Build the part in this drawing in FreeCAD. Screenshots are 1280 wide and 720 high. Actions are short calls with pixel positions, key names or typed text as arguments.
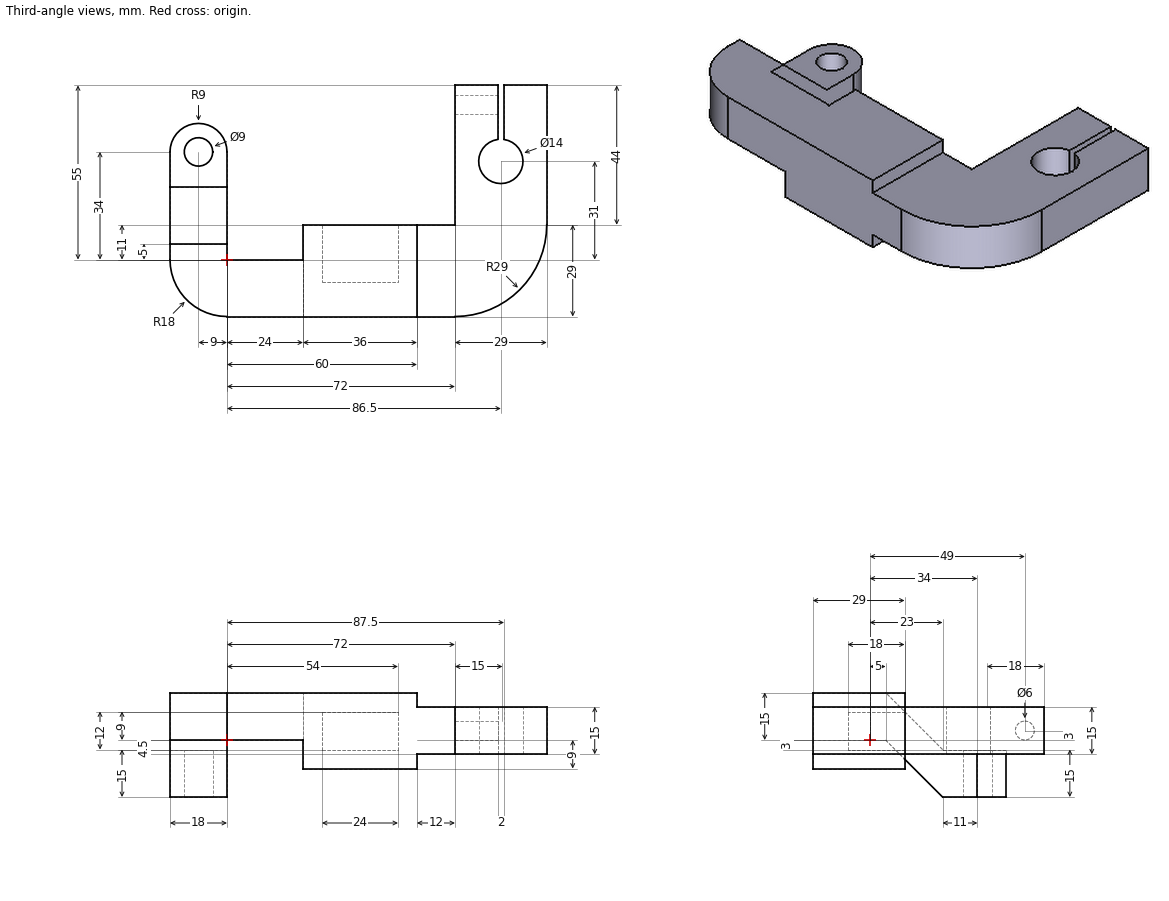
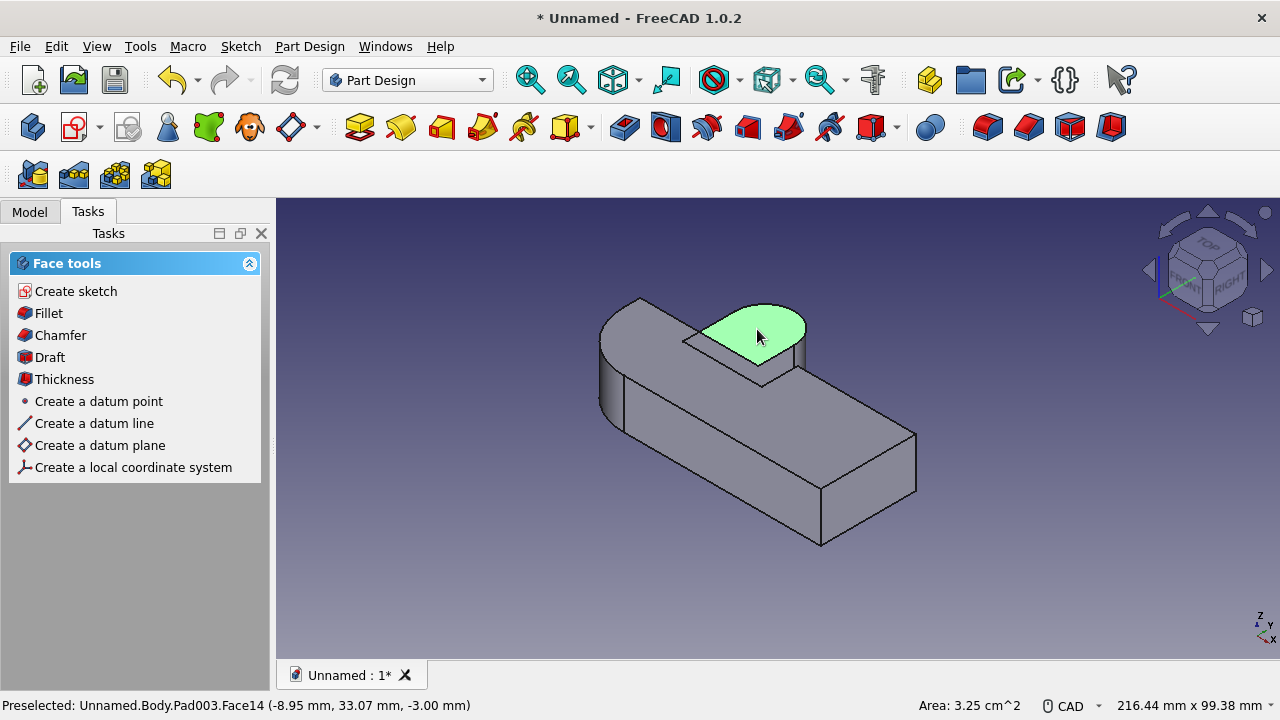
click(74, 128)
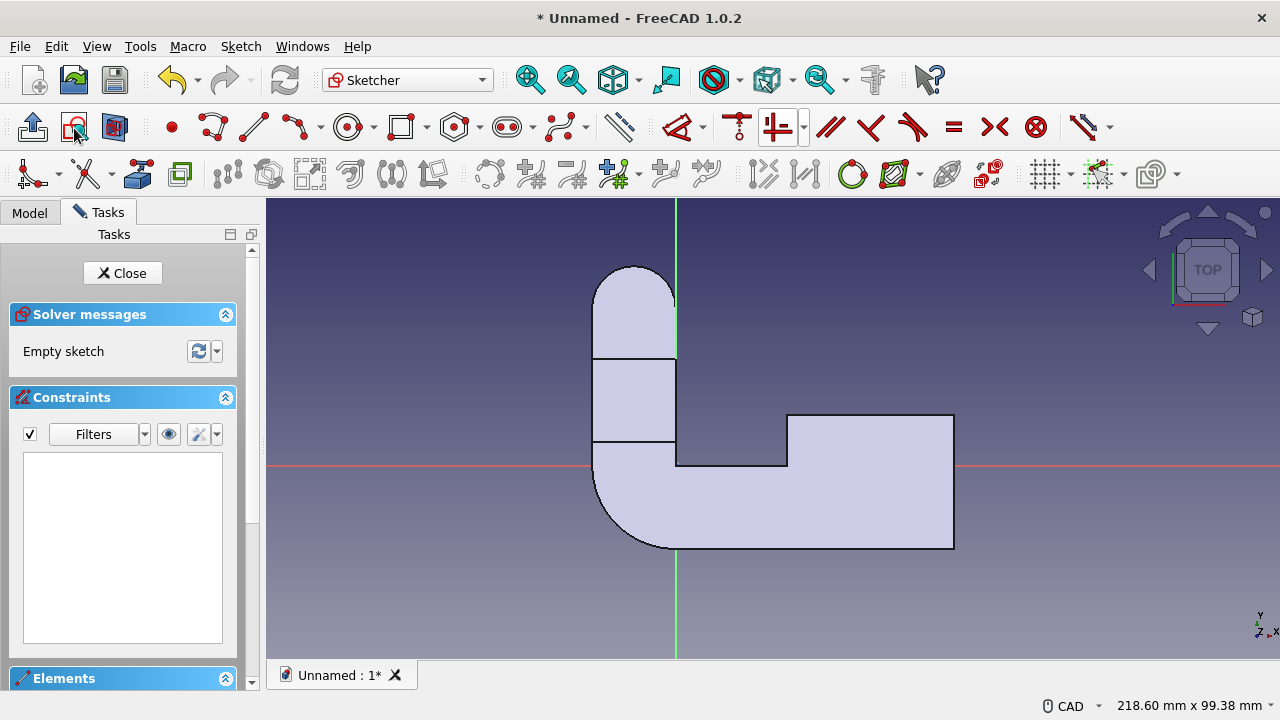
scroll(623, 289, up, 10)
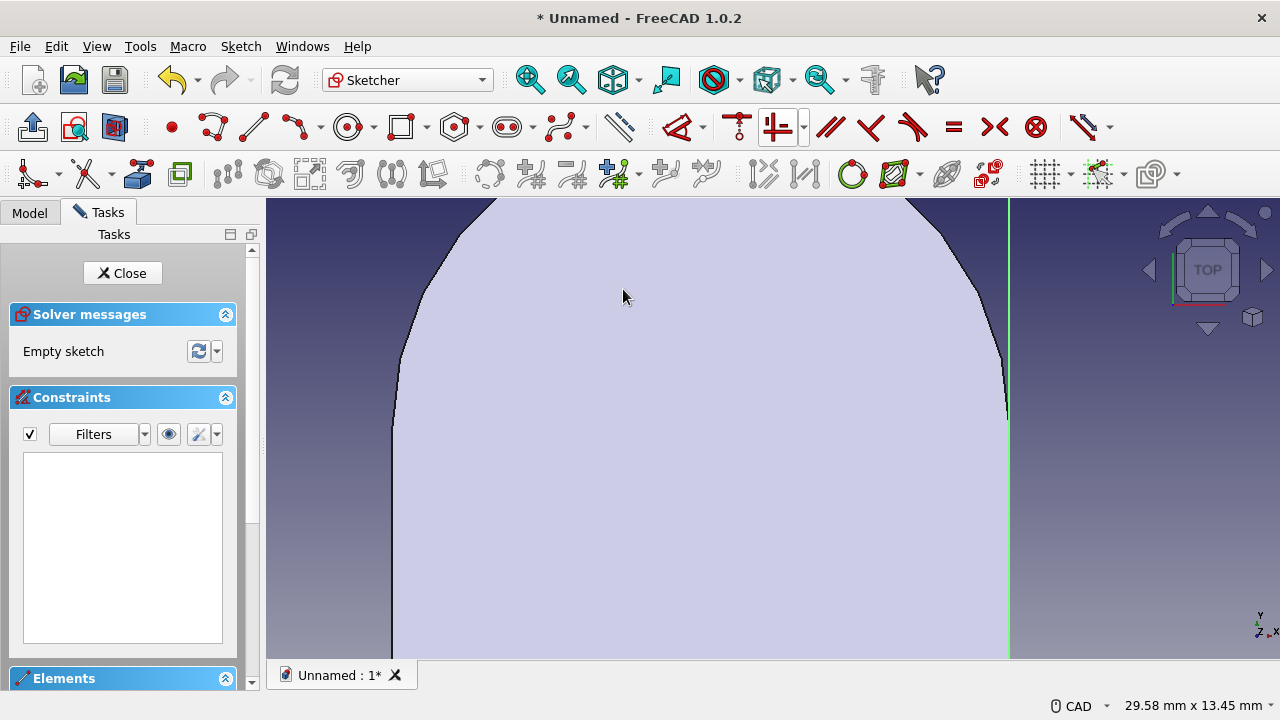
click(348, 128)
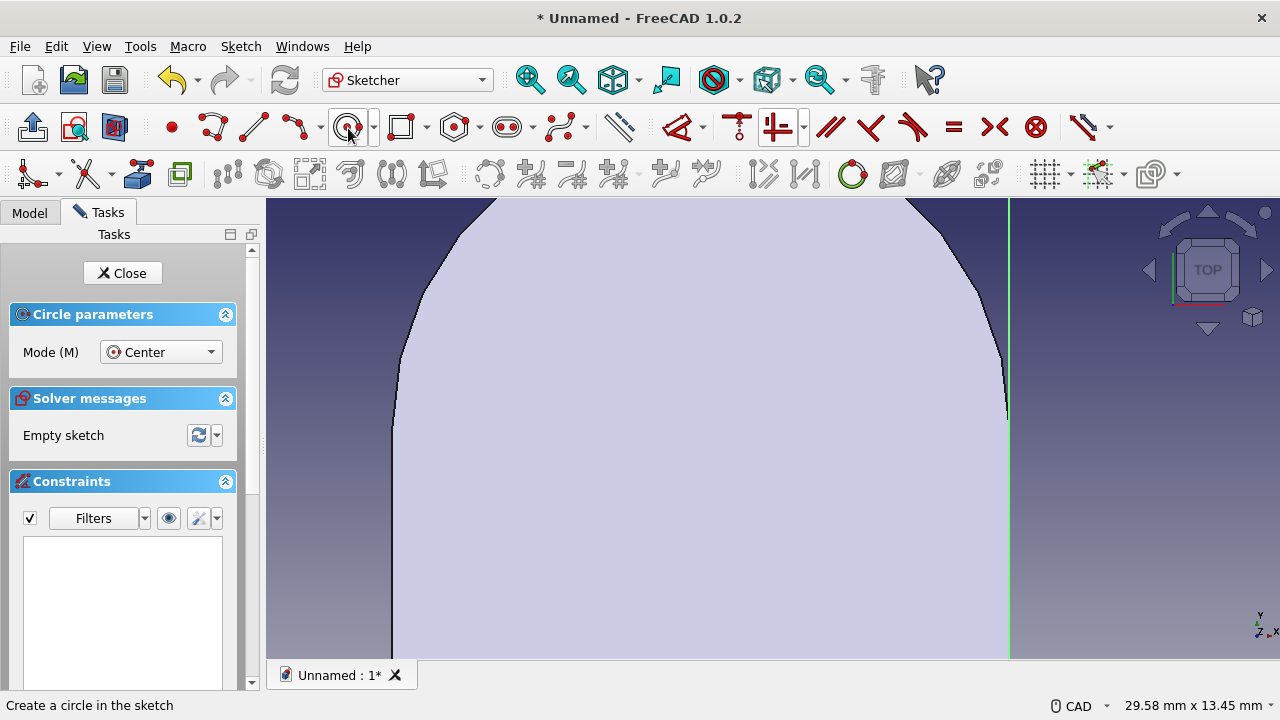
click(701, 427)
move(810, 318)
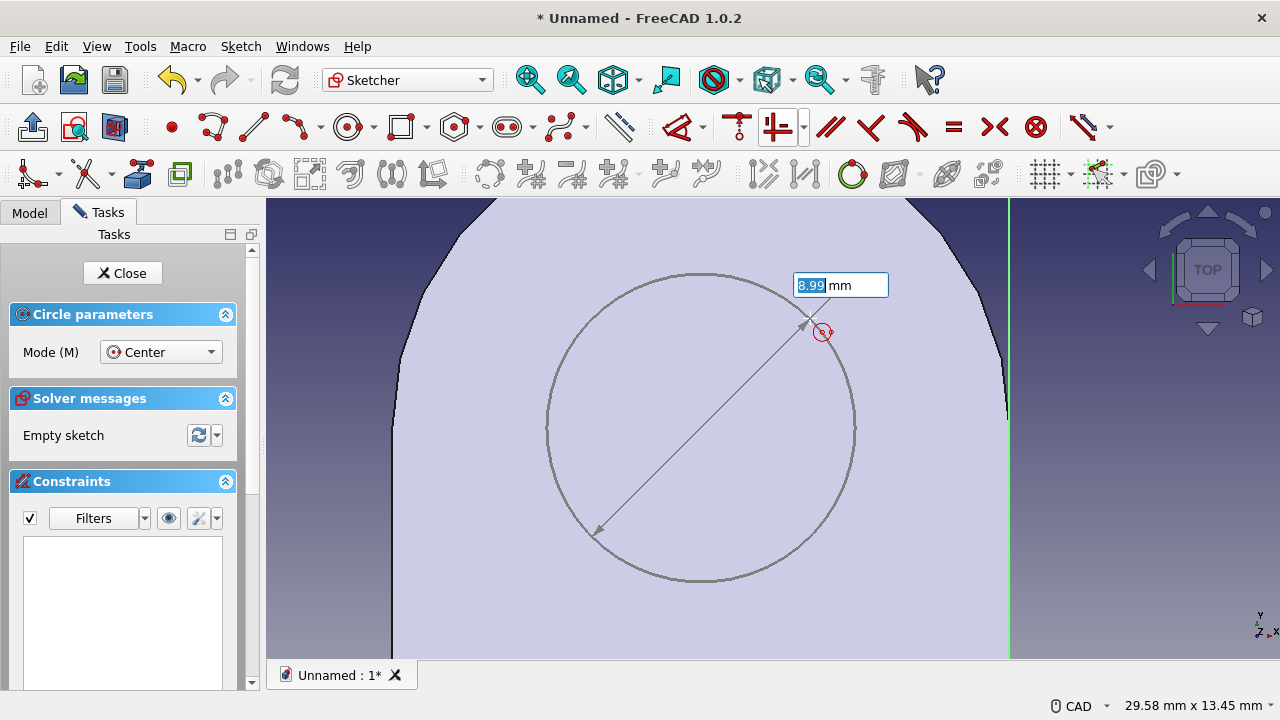
text(9)
key(Return)
key(Escape)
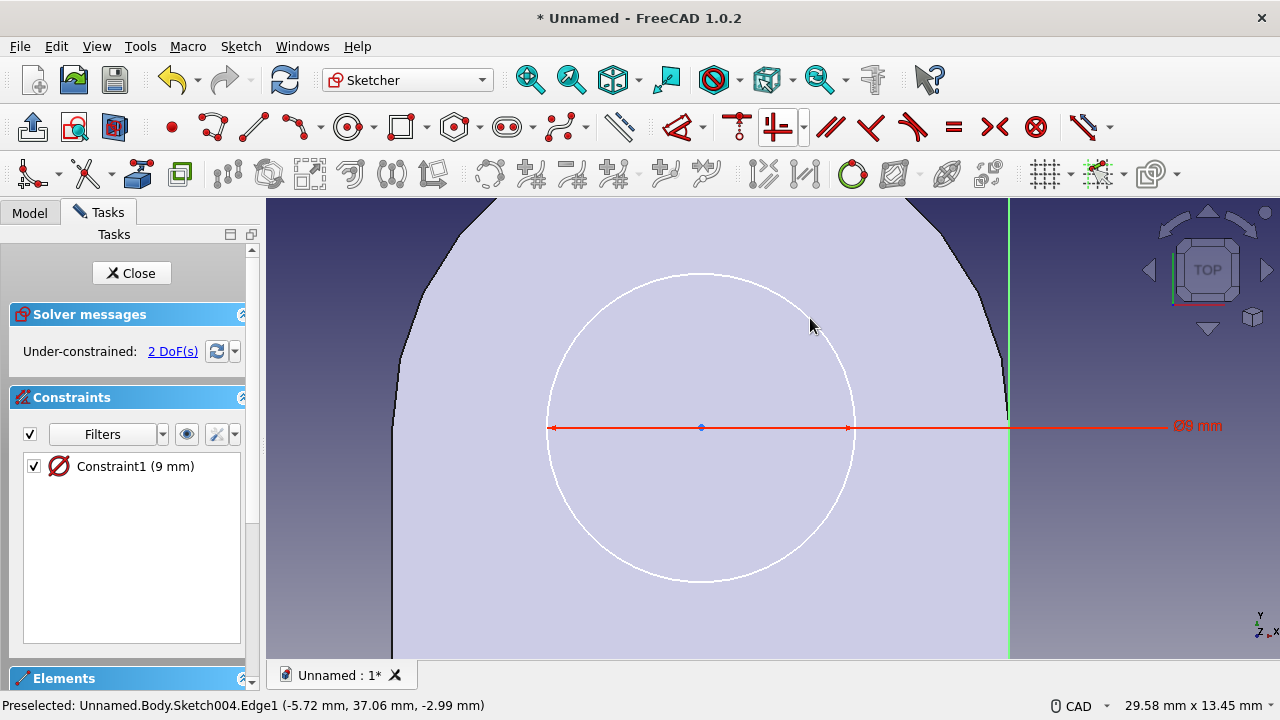
click(676, 128)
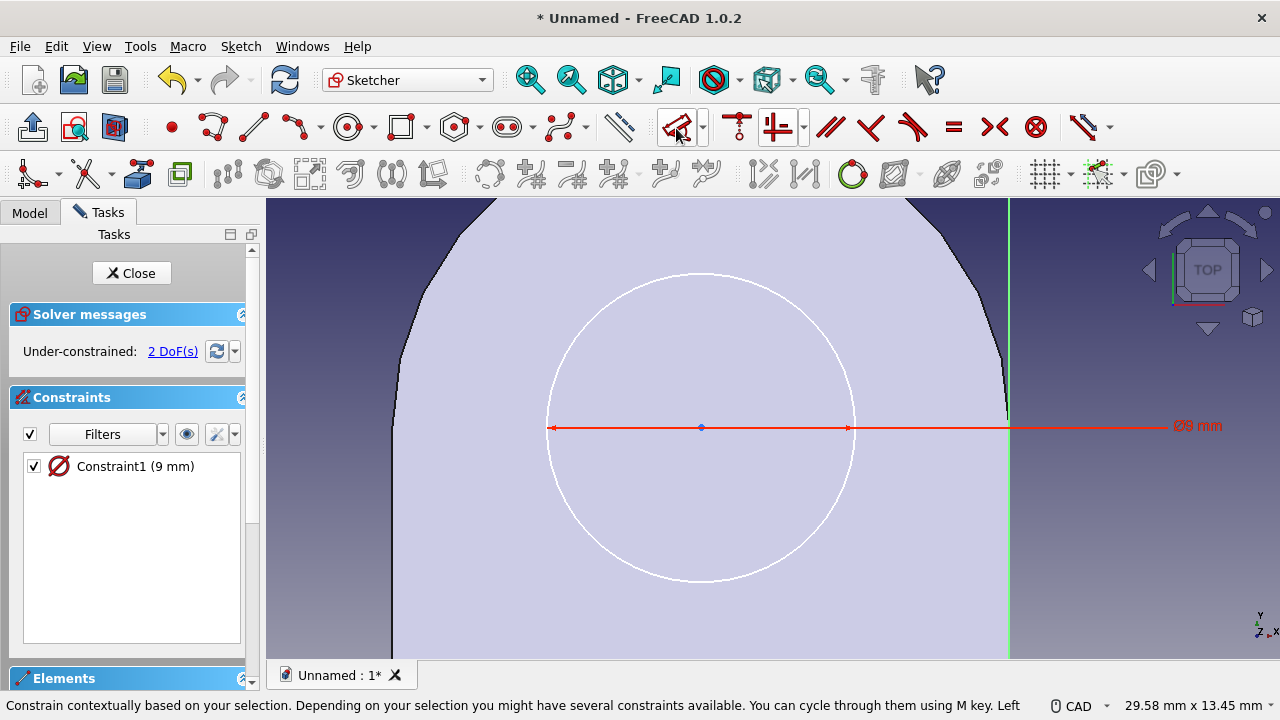
click(701, 428)
click(784, 394)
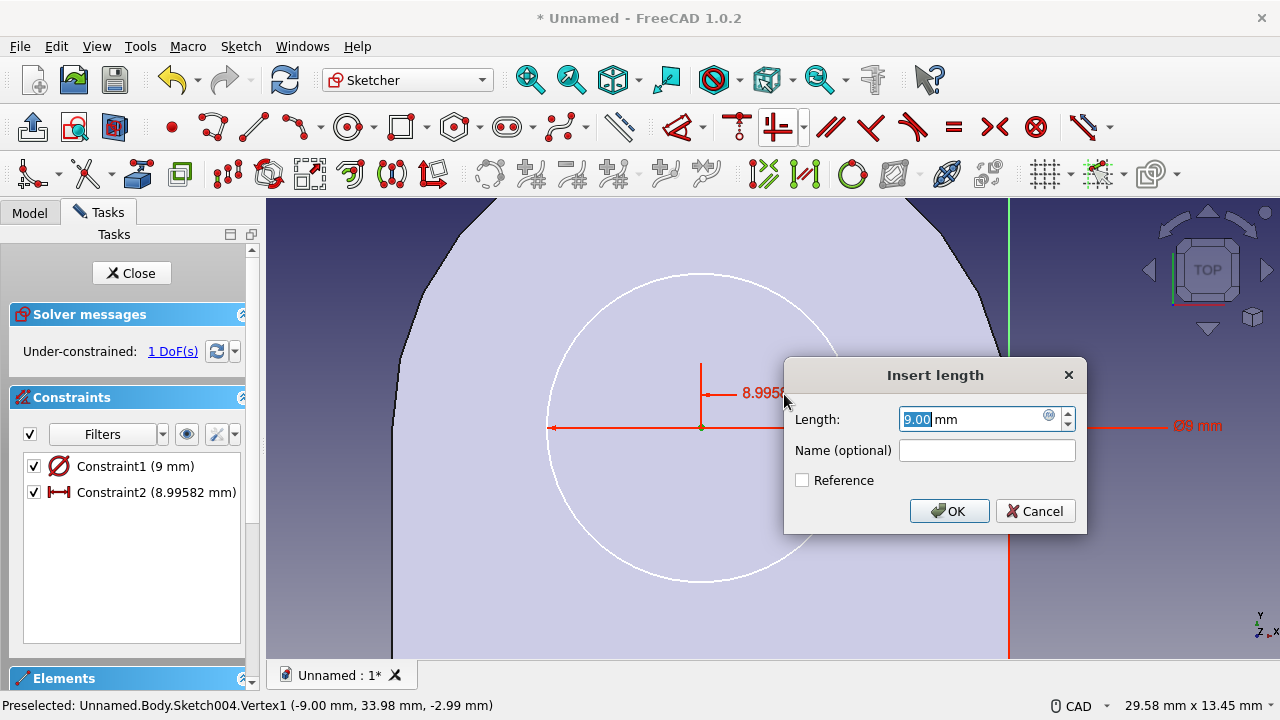
text(9)
key(Return)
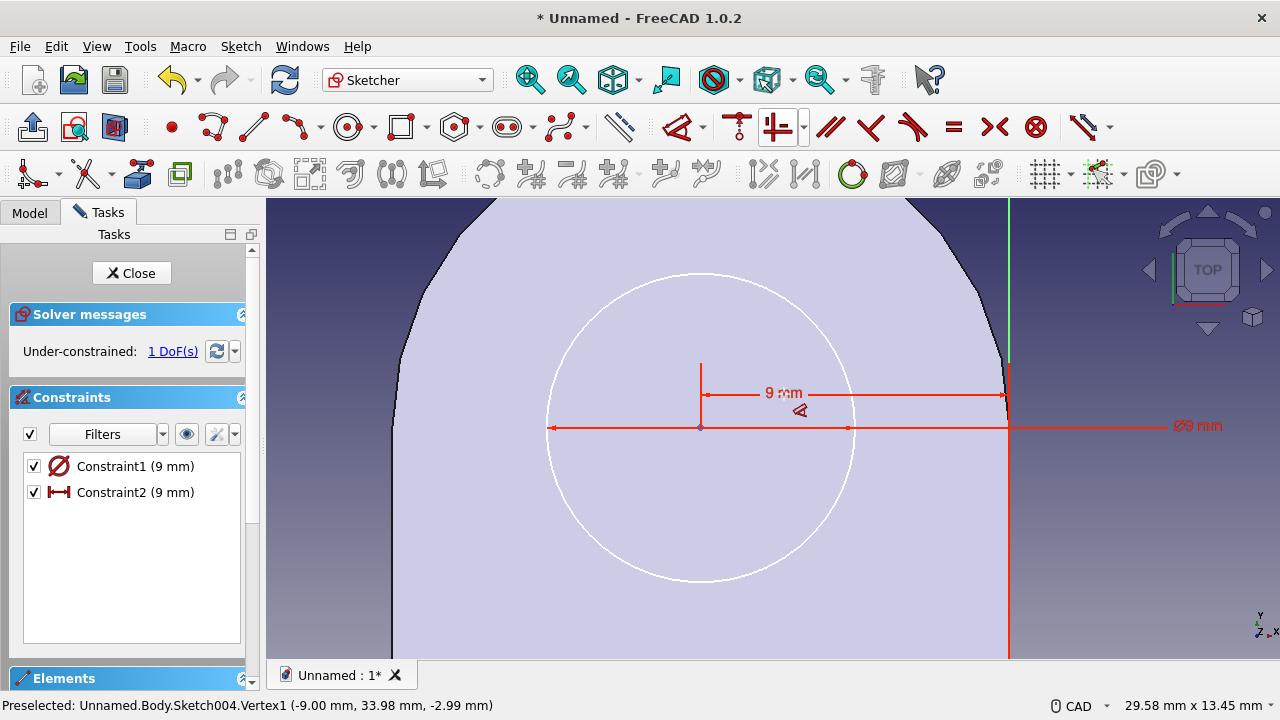
click(701, 428)
click(1043, 530)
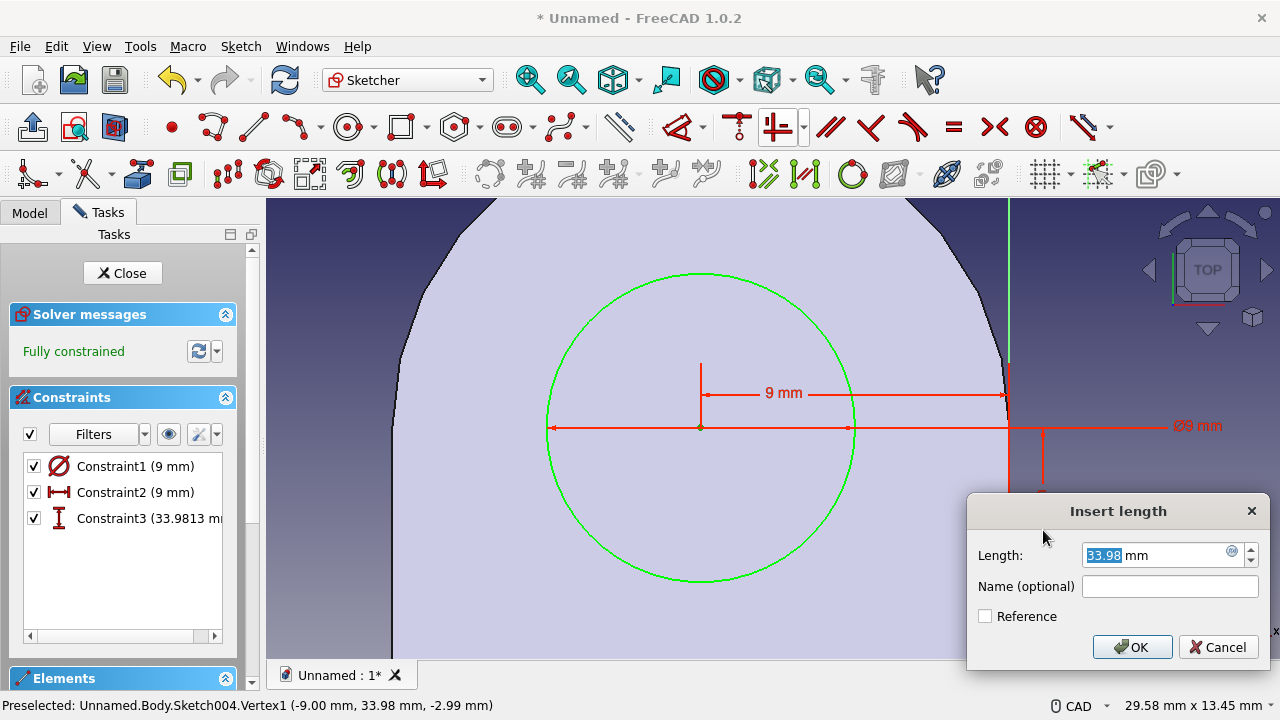
text(34)
key(Return)
key(Escape)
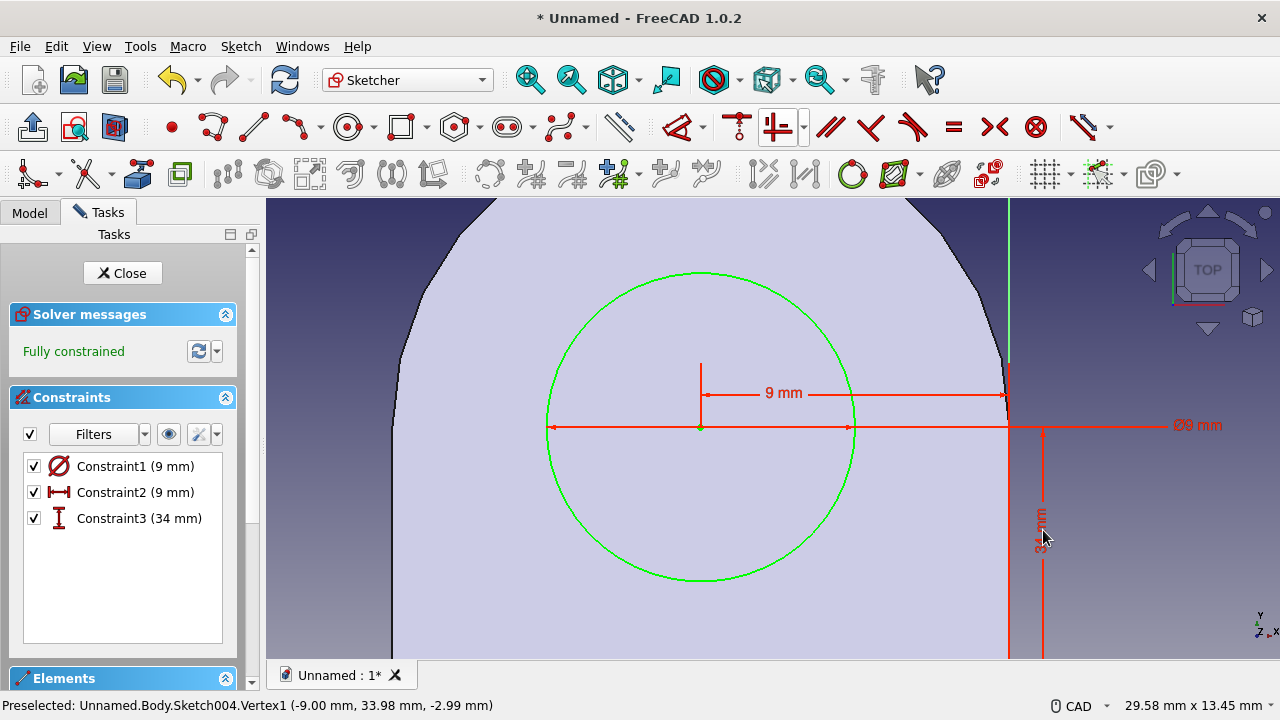
click(123, 273)